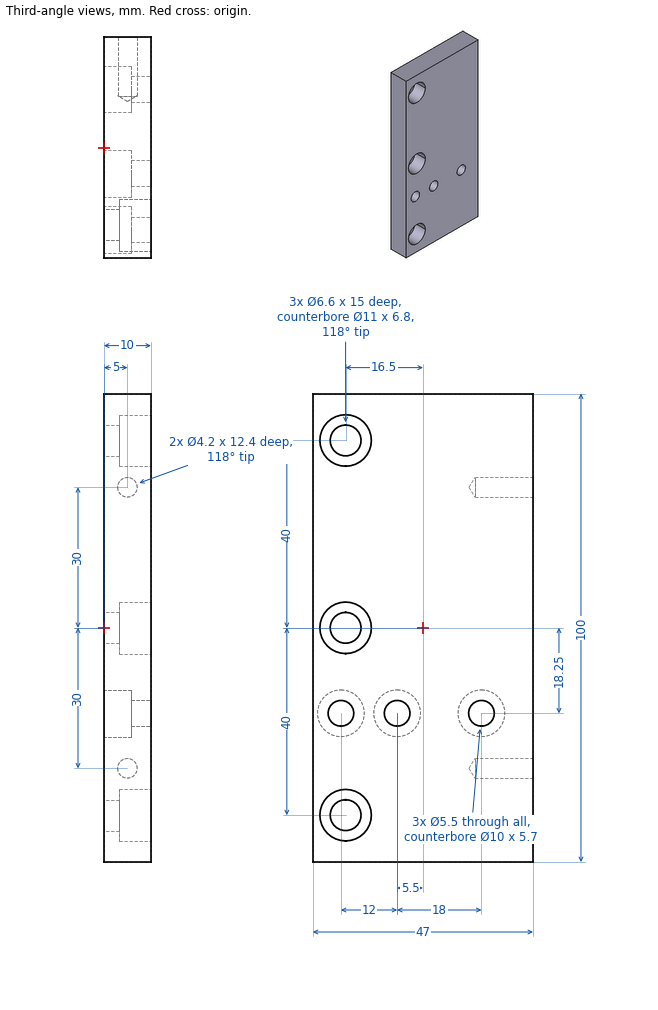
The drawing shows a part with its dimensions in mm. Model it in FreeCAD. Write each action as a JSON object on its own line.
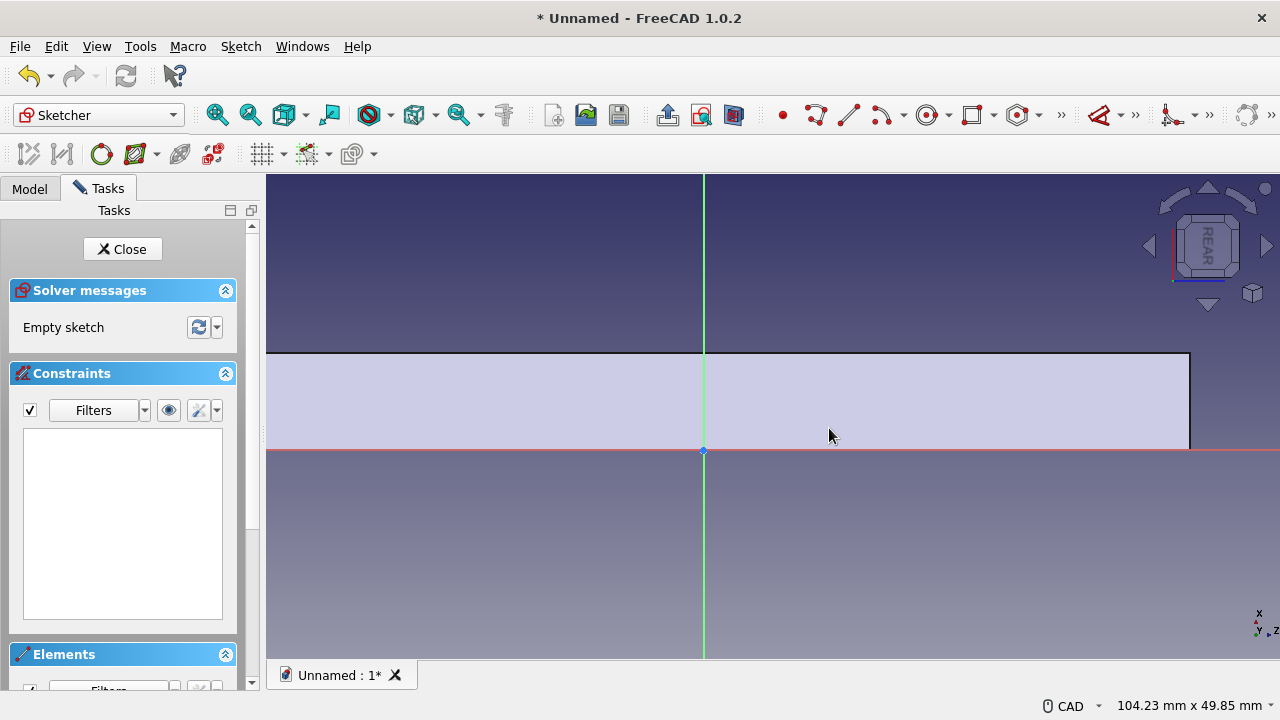
{"action": "left_click", "coordinate": [926, 116]}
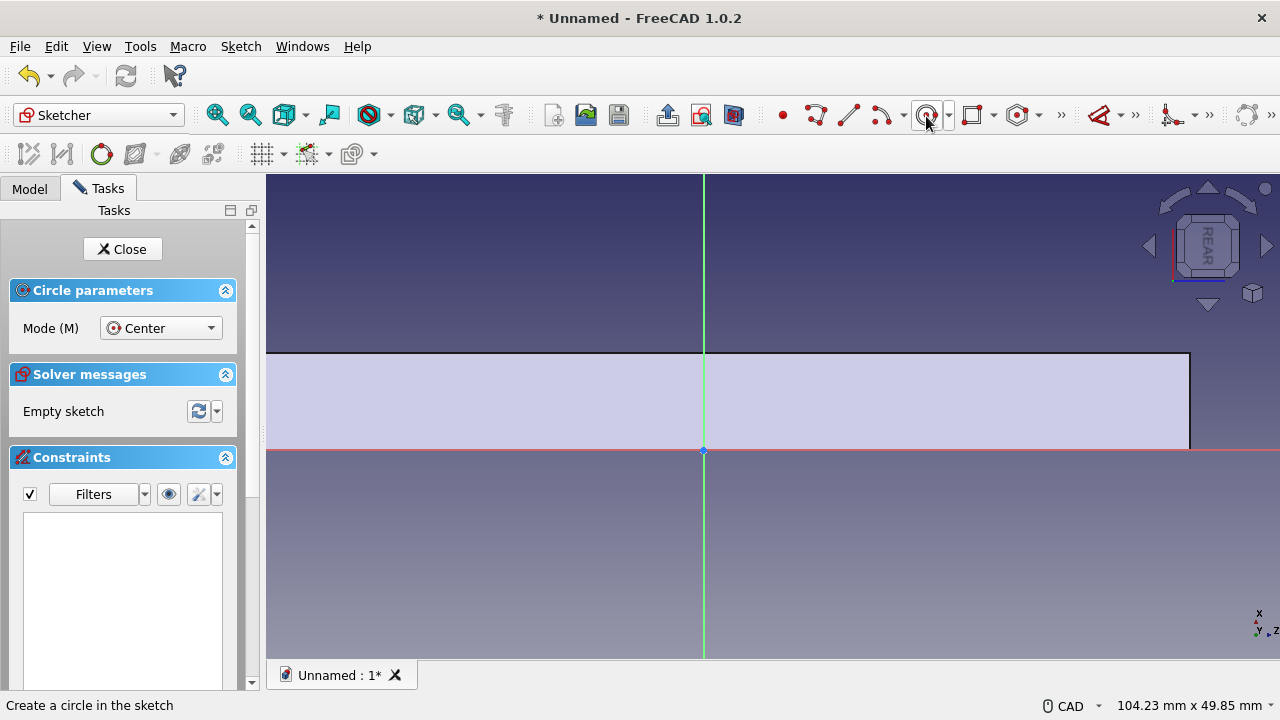
{"action": "left_click", "coordinate": [996, 402]}
{"action": "mouse_move", "coordinate": [1010, 387]}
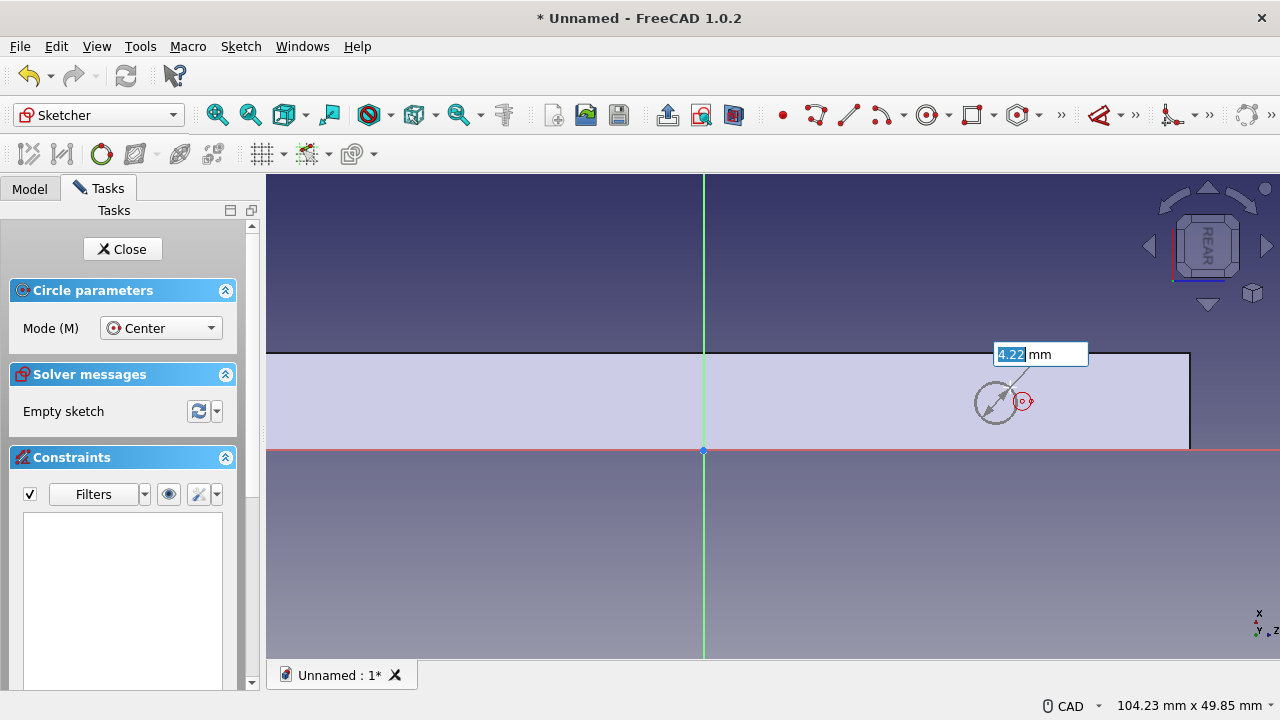
{"action": "type", "text": "4.2"}
{"action": "key", "text": "Return"}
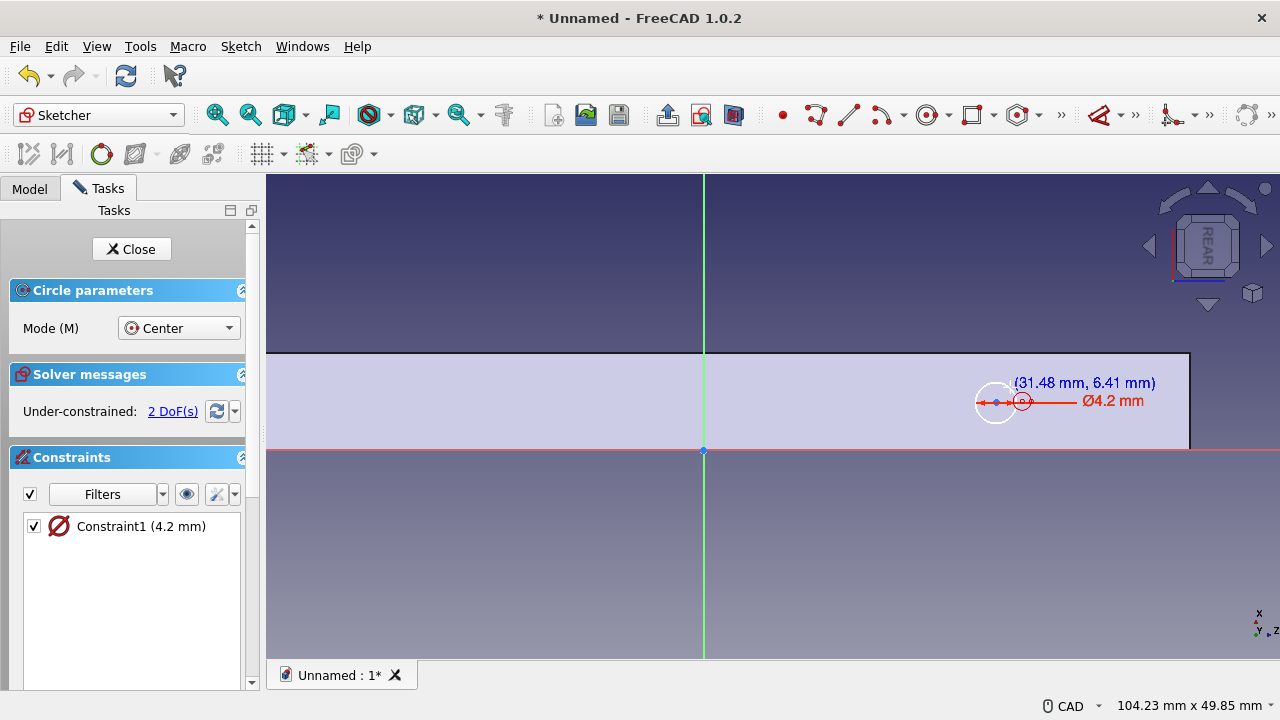
{"action": "left_click", "coordinate": [412, 402]}
{"action": "mouse_move", "coordinate": [426, 387]}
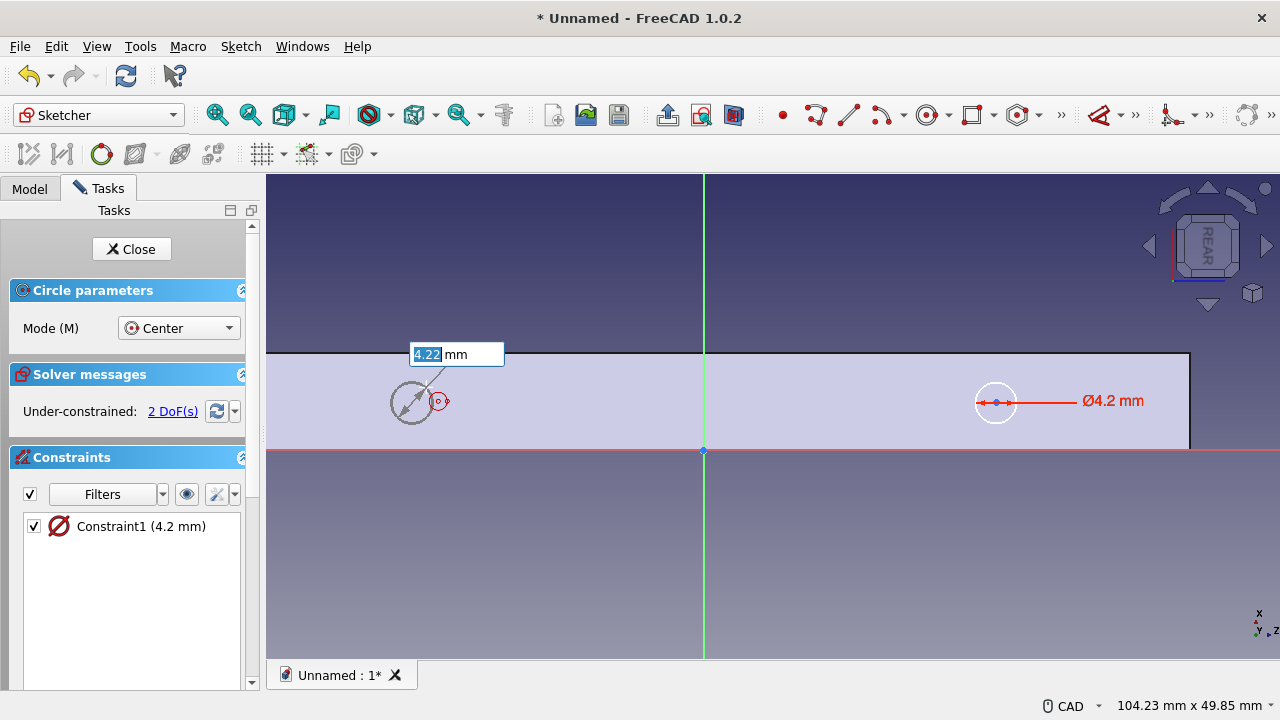
{"action": "type", "text": "4.2"}
{"action": "key", "text": "Return"}
{"action": "key", "text": "Escape"}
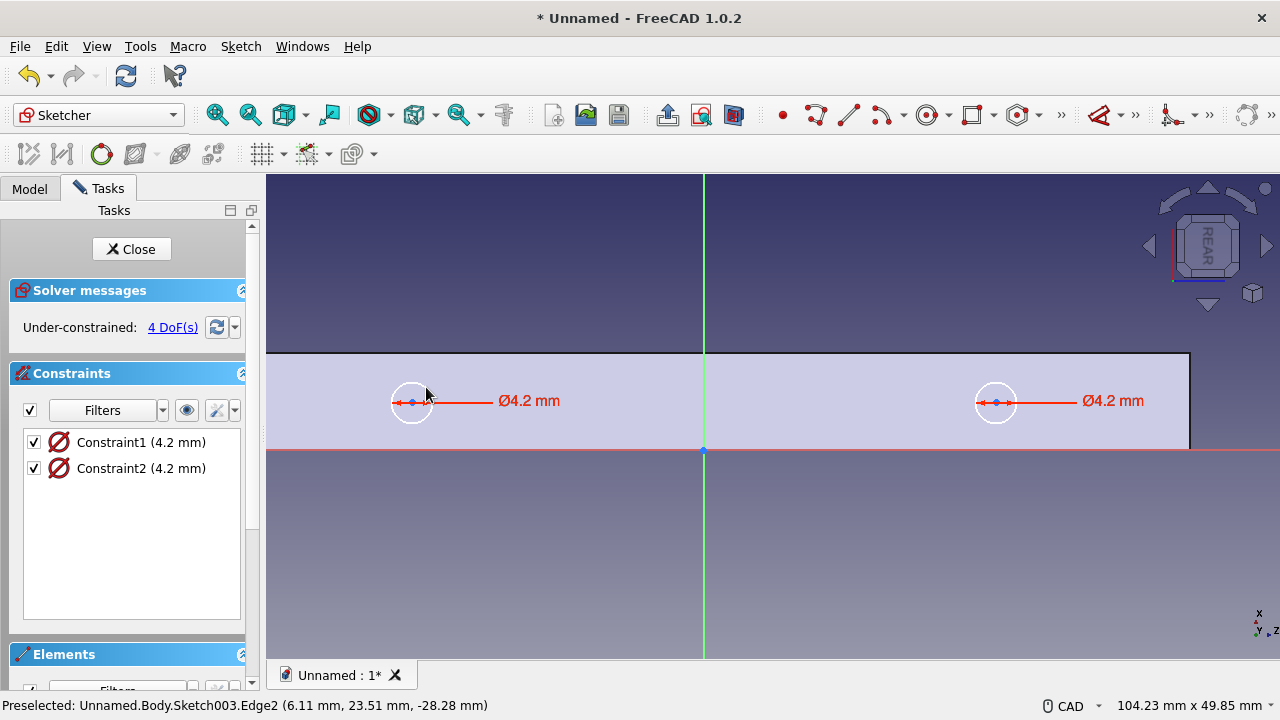
{"action": "left_click", "coordinate": [996, 403]}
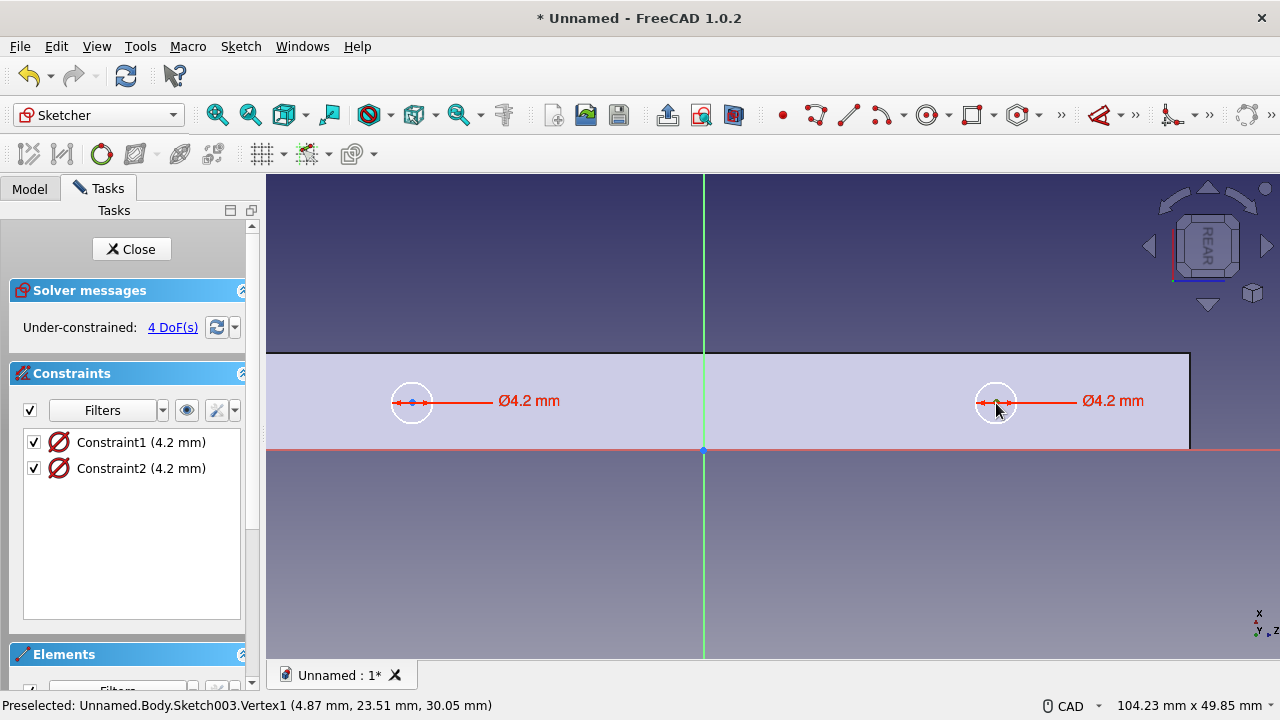
{"action": "left_click", "coordinate": [412, 403]}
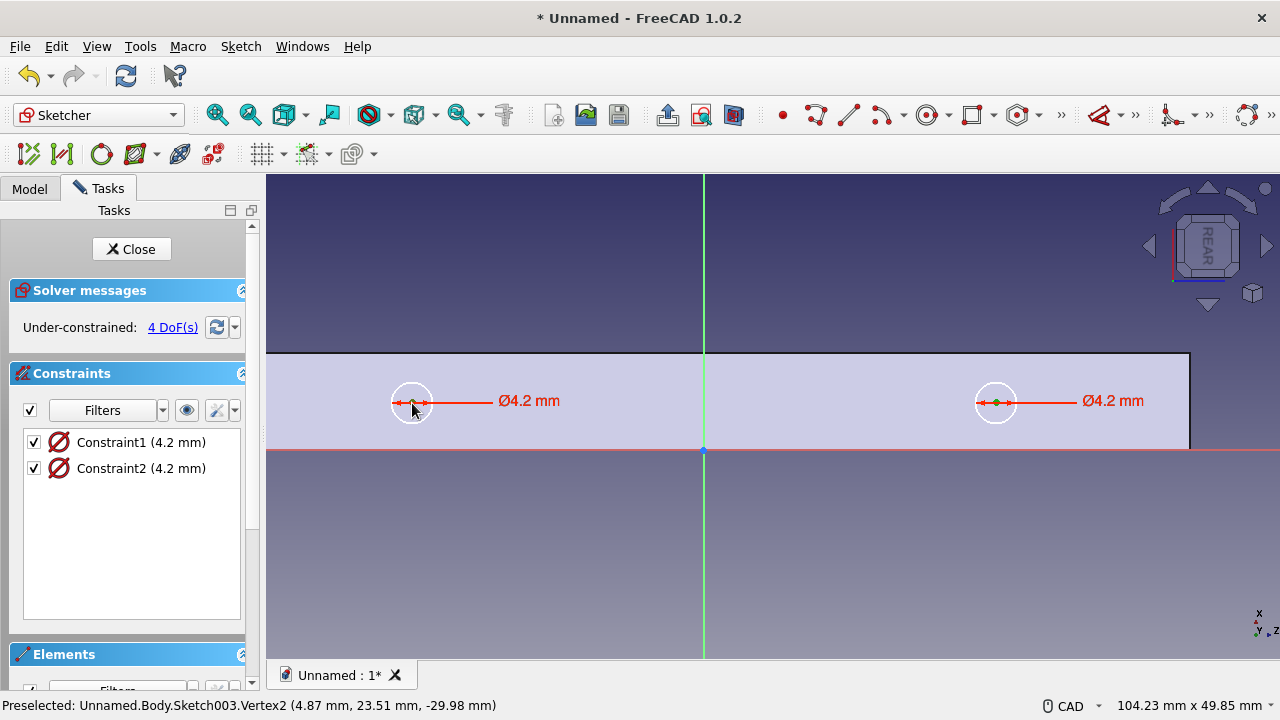
{"action": "key", "text": "h"}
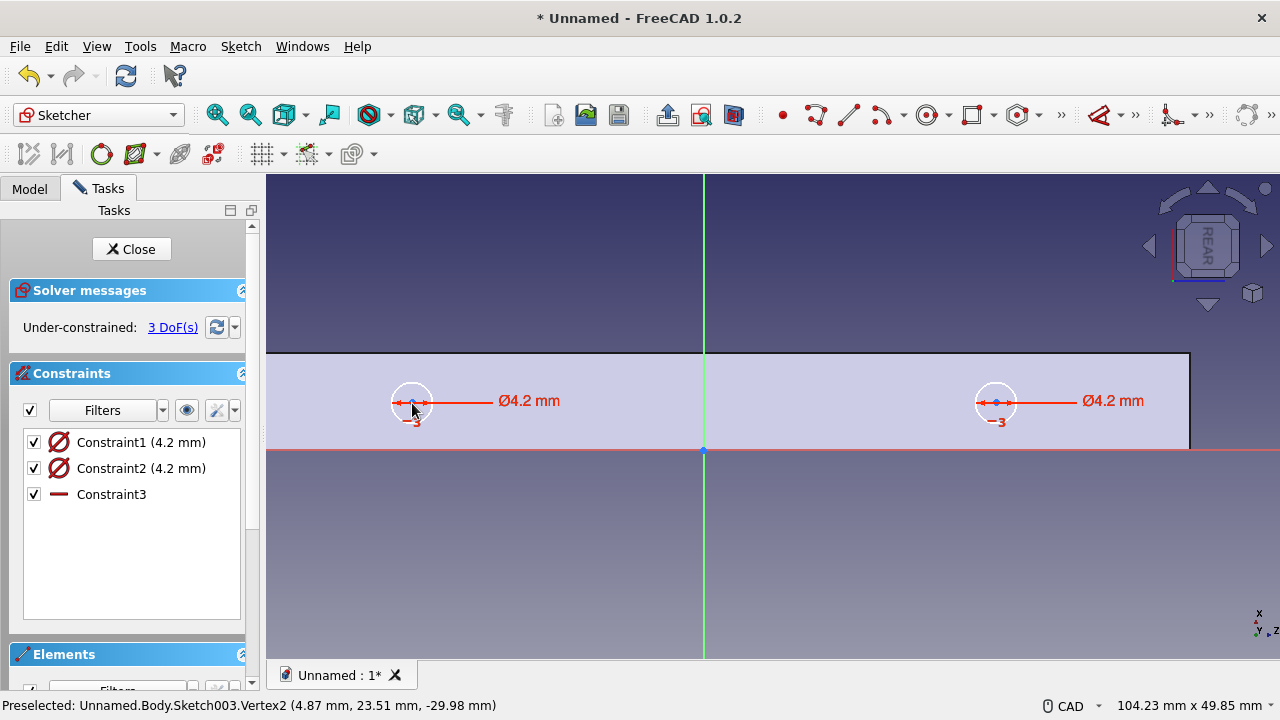
{"action": "left_click", "coordinate": [1098, 116]}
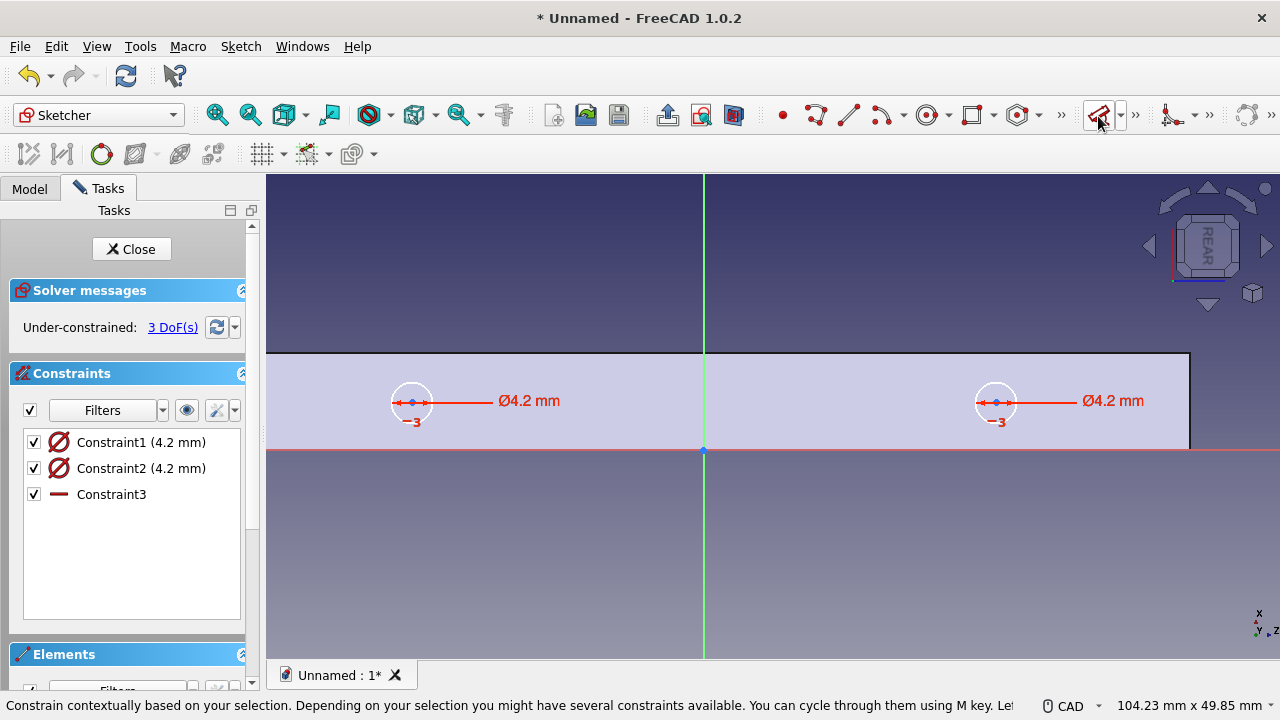
{"action": "left_click", "coordinate": [996, 403]}
{"action": "left_click", "coordinate": [1030, 427]}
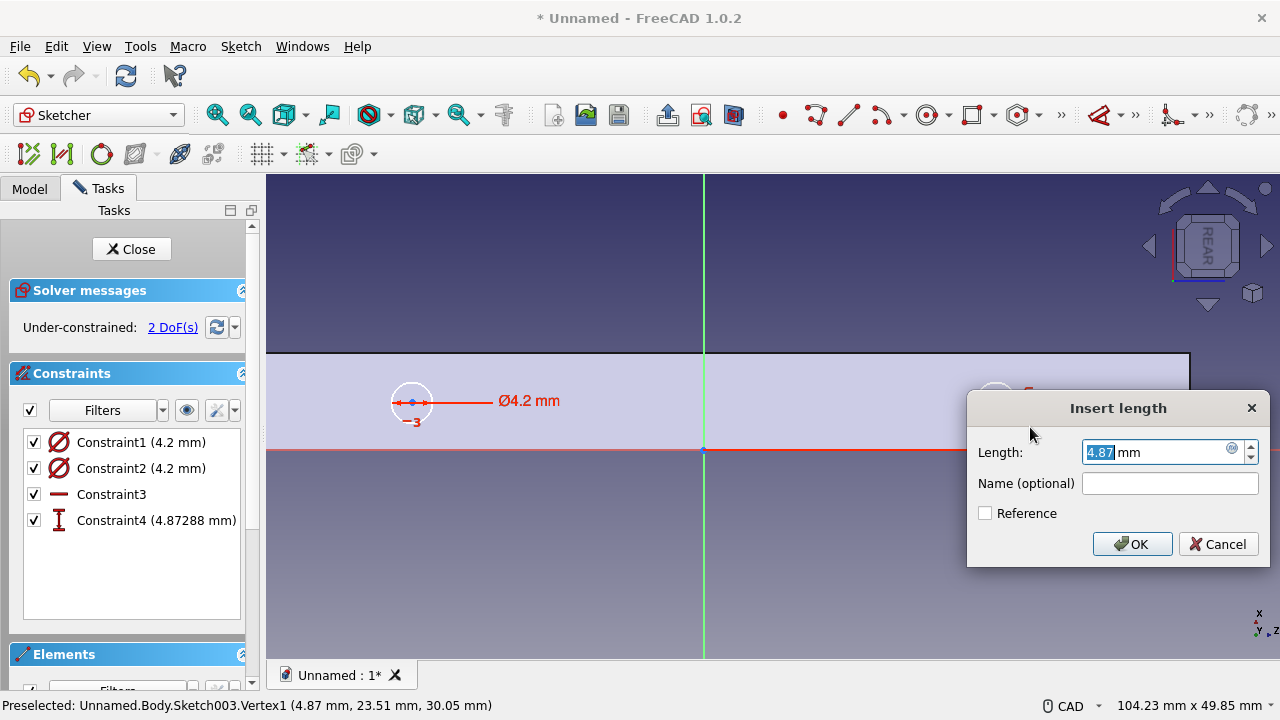
{"action": "type", "text": "5"}
{"action": "key", "text": "Return"}